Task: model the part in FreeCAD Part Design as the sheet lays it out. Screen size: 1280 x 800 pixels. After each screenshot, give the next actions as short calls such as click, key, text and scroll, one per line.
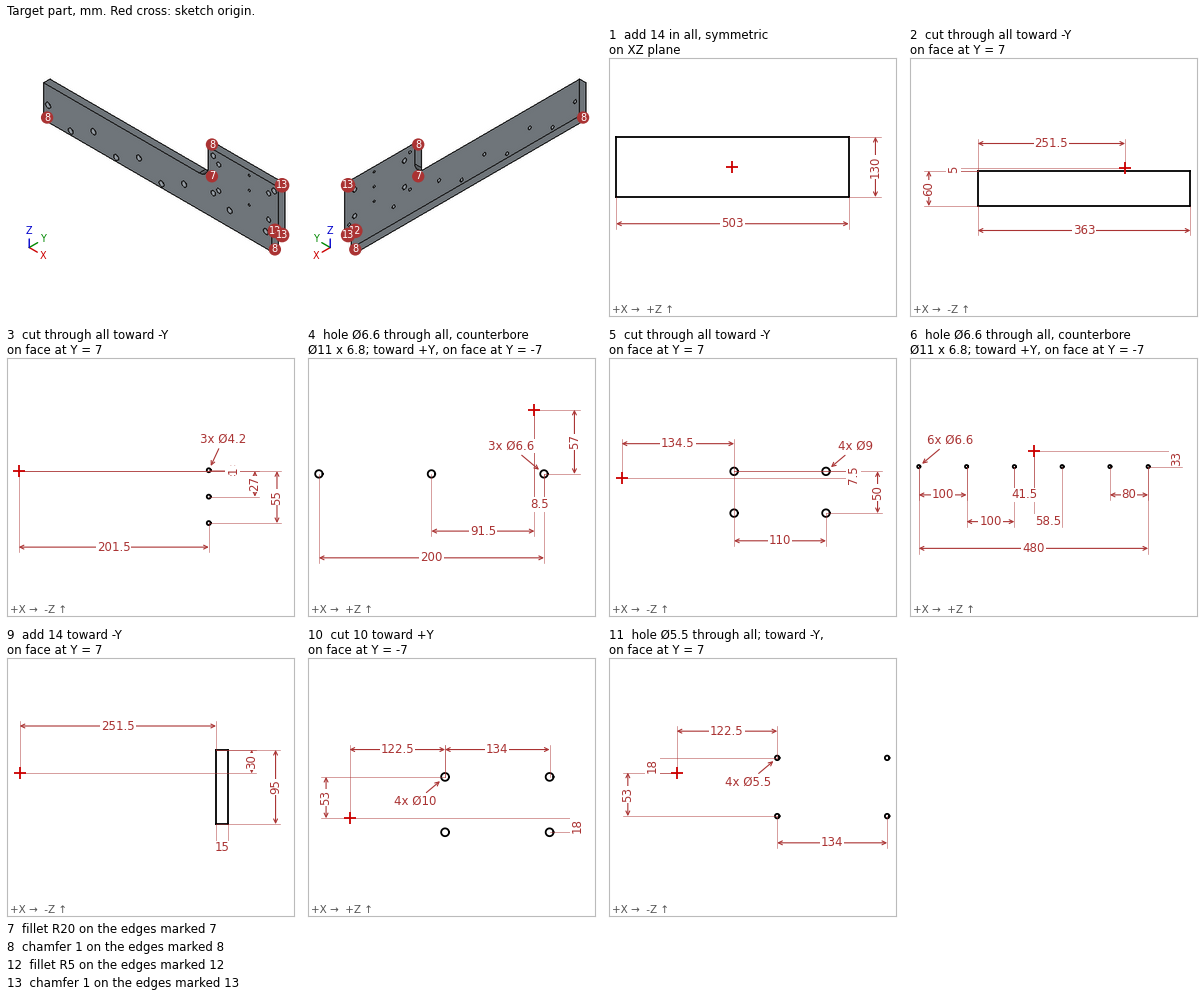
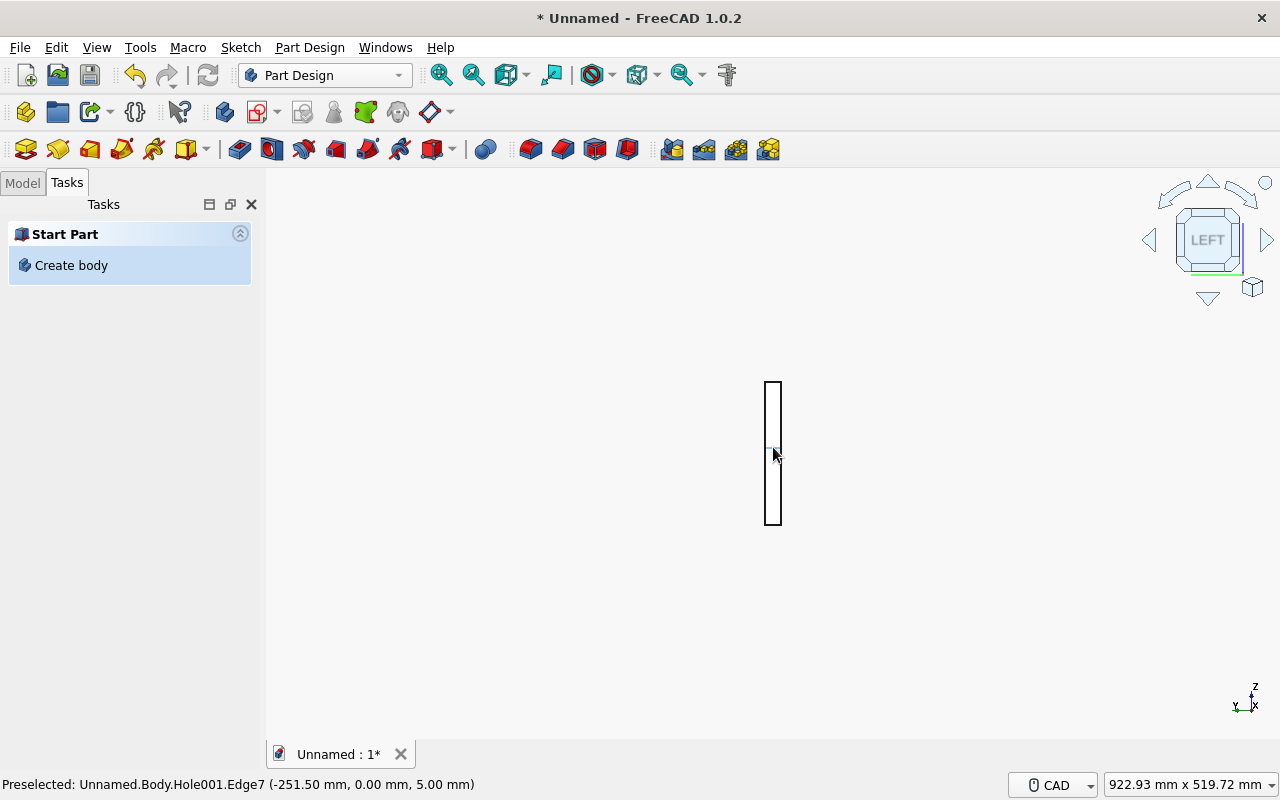
key(v)
key(3)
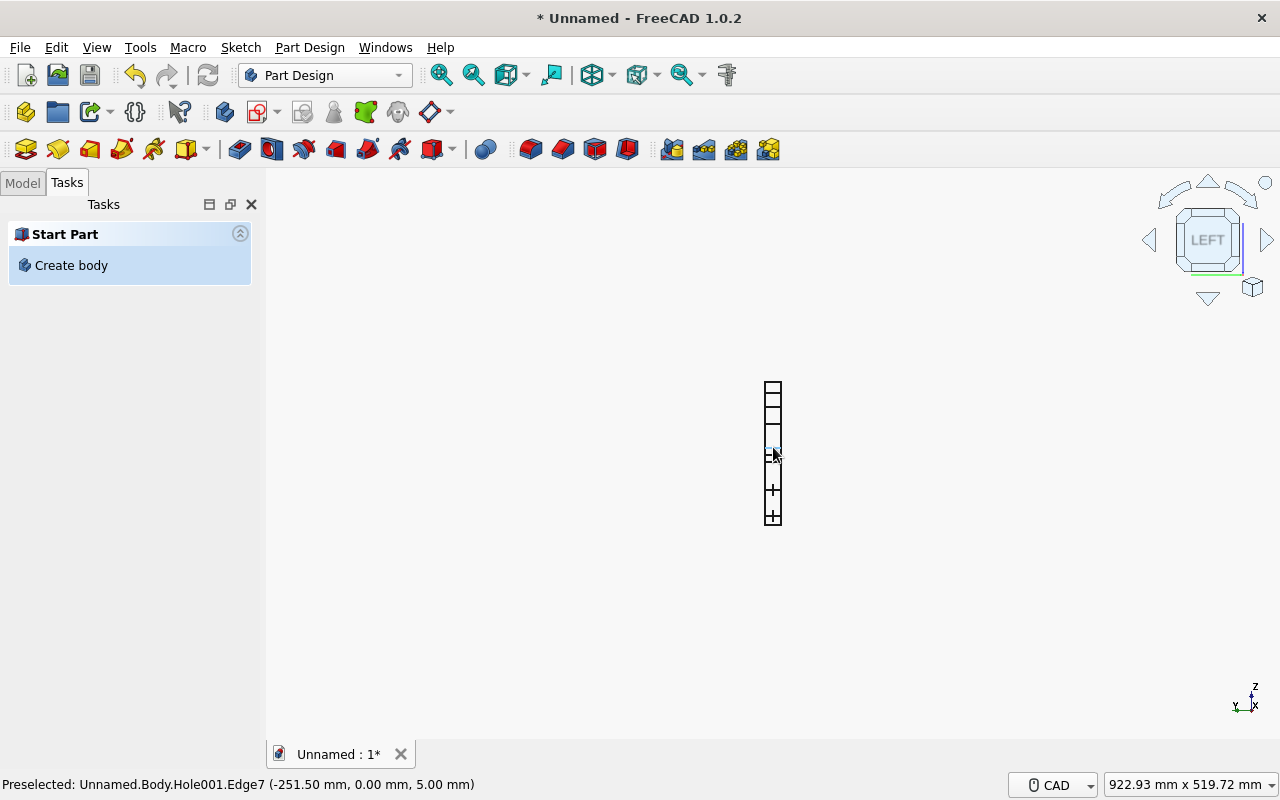
key(0)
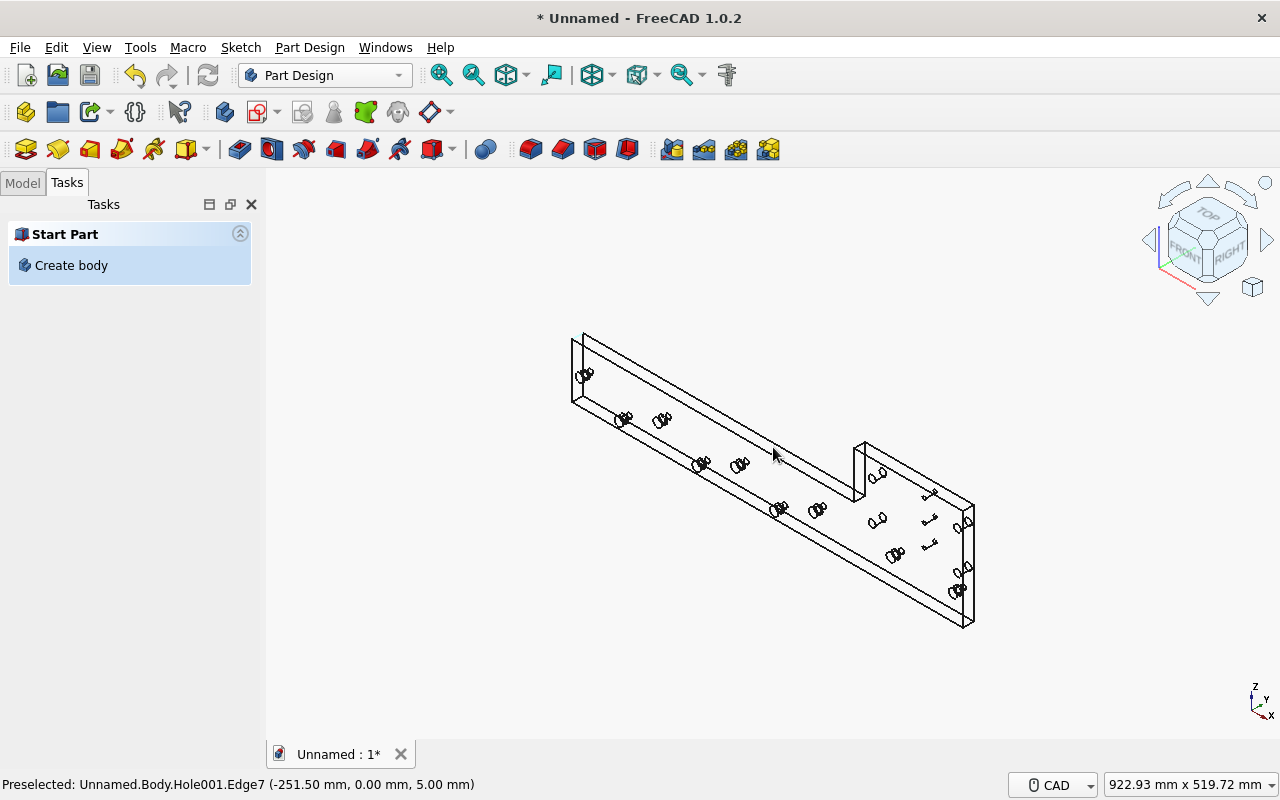
click(861, 497)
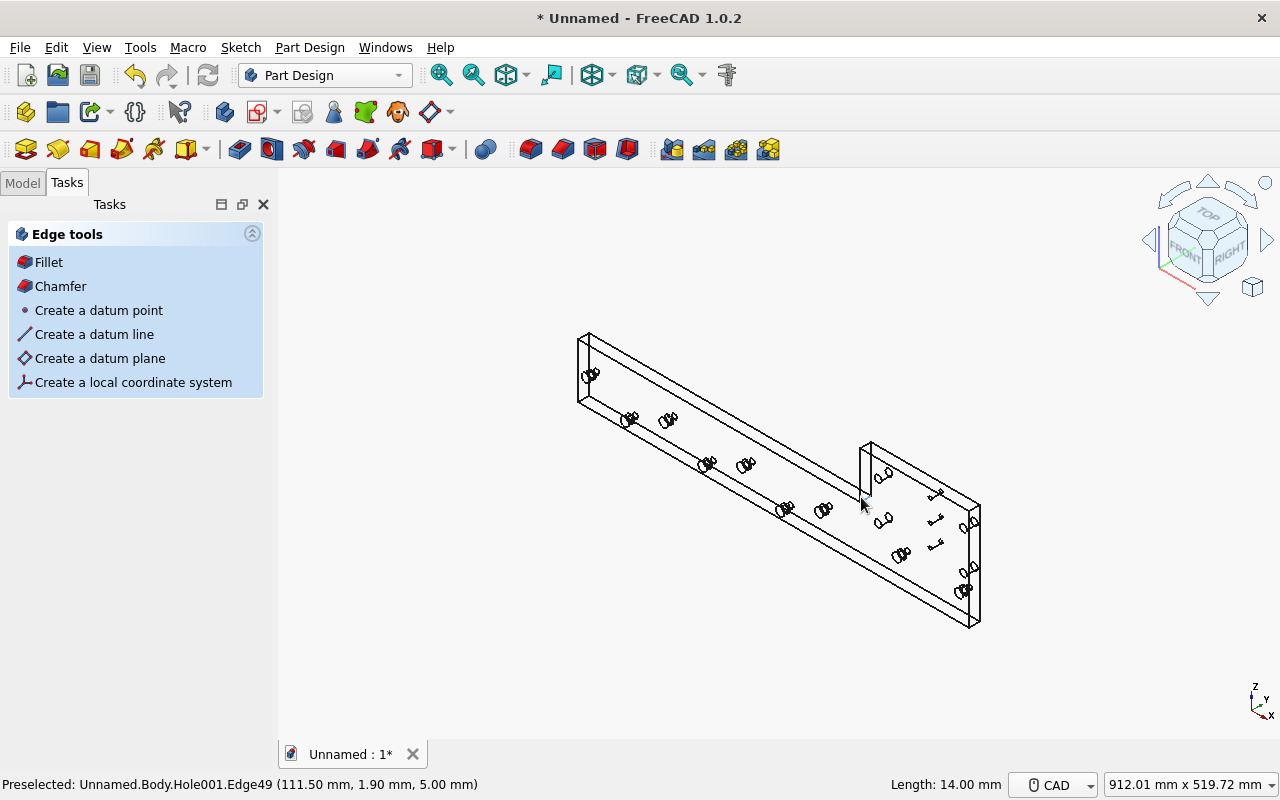
key(v)
key(1)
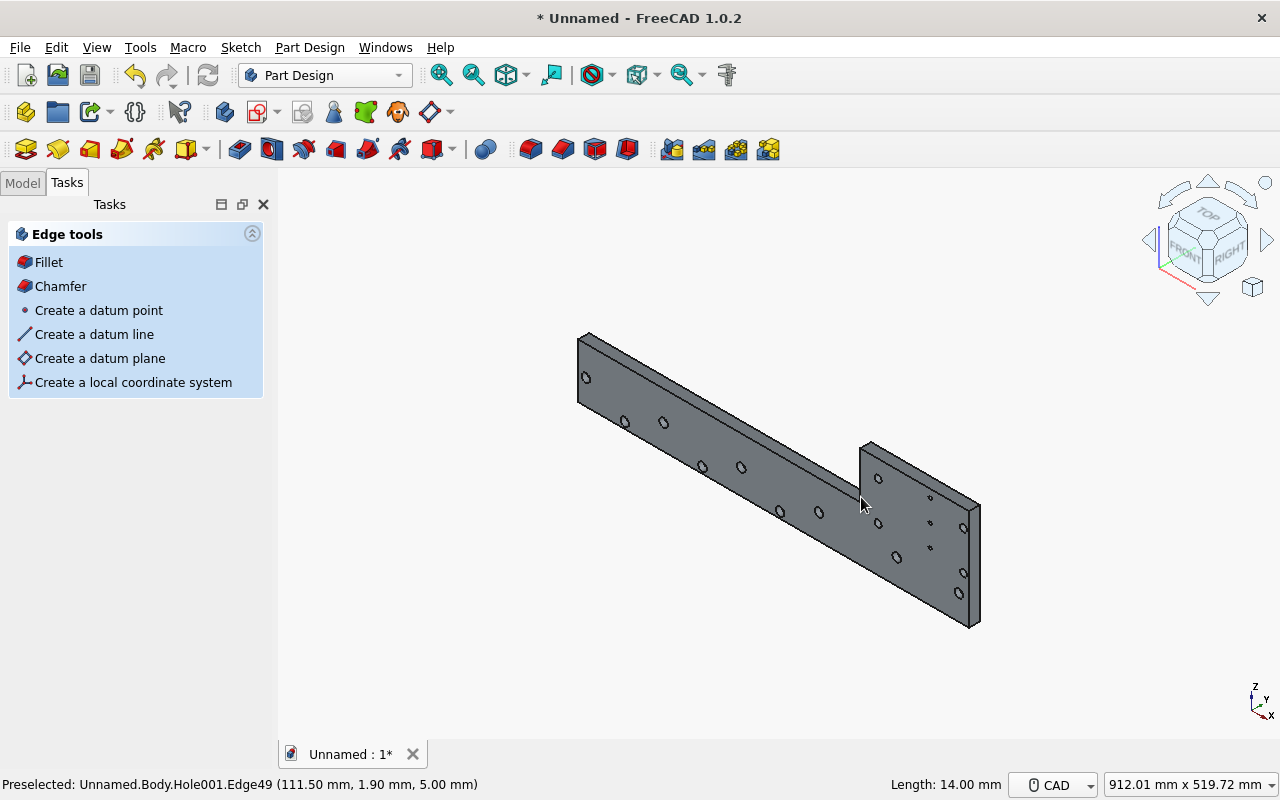
click(532, 150)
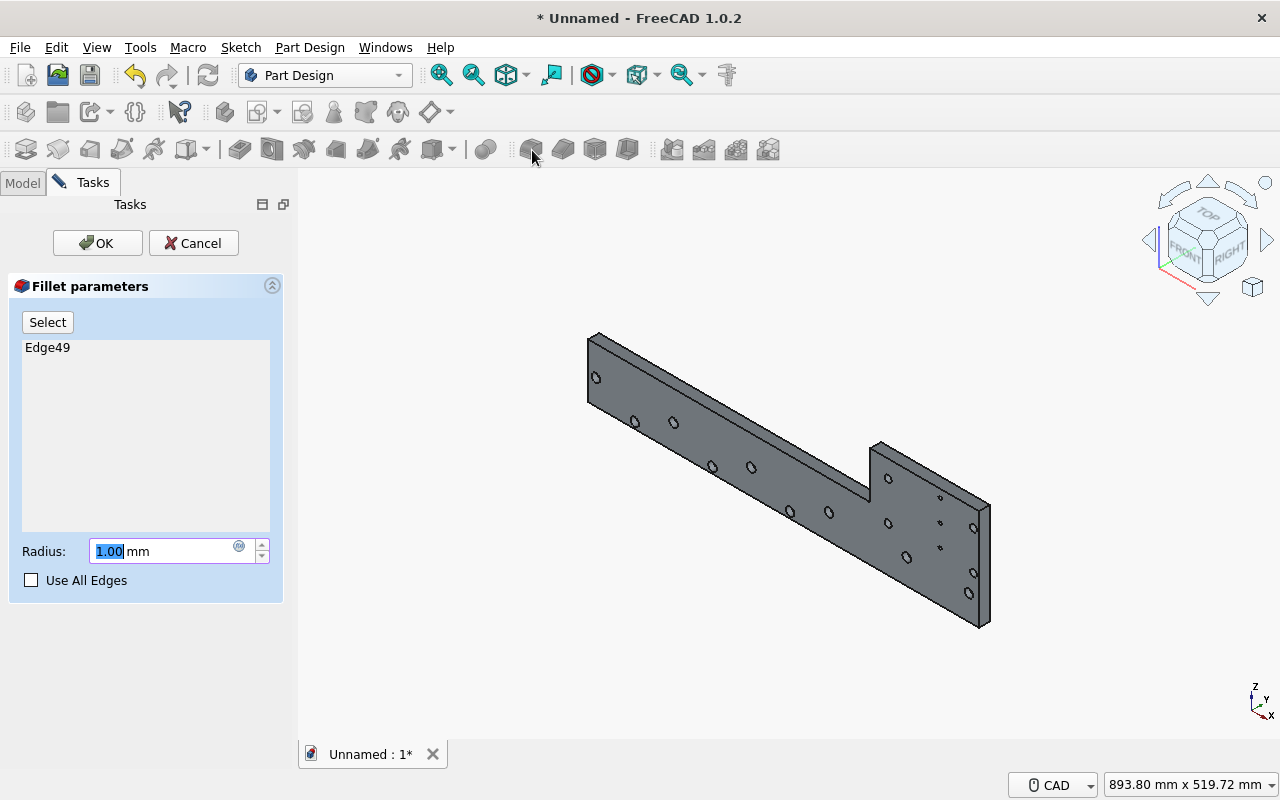
text(20)
key(Tab)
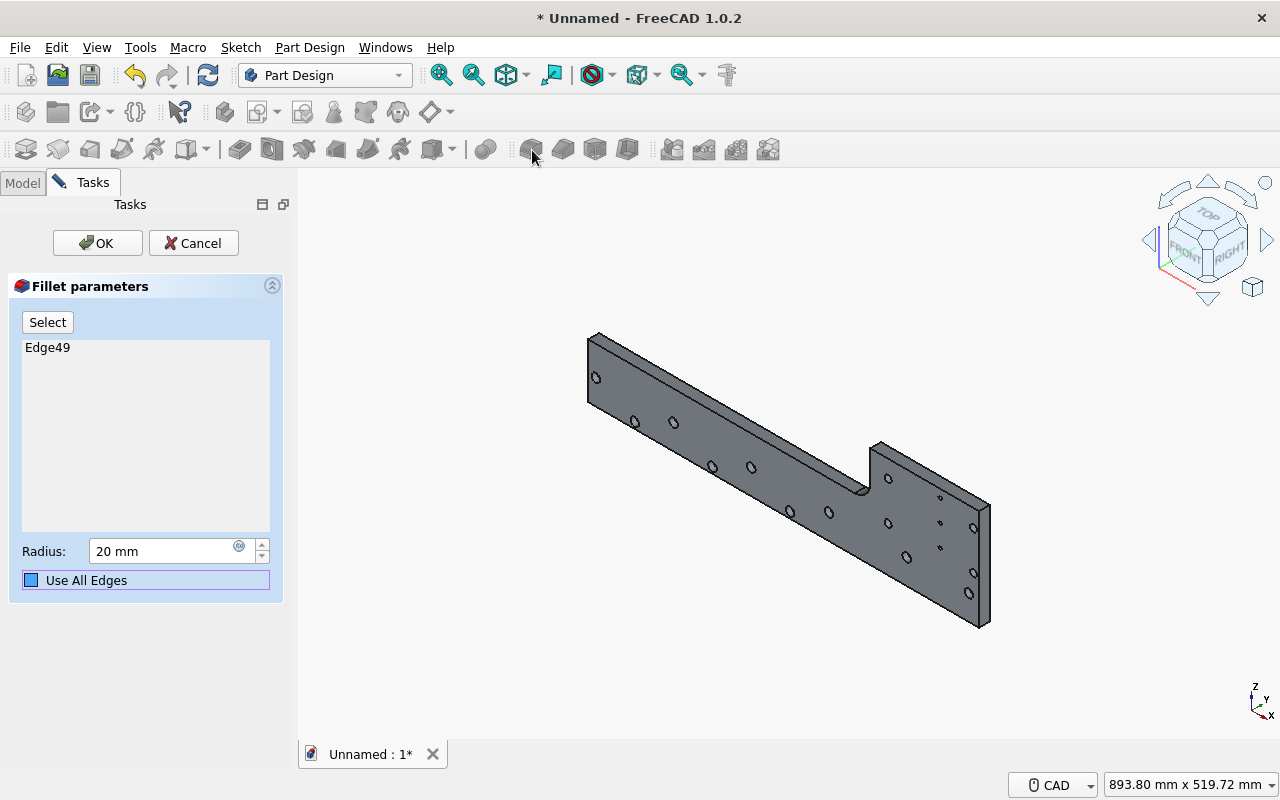
click(98, 243)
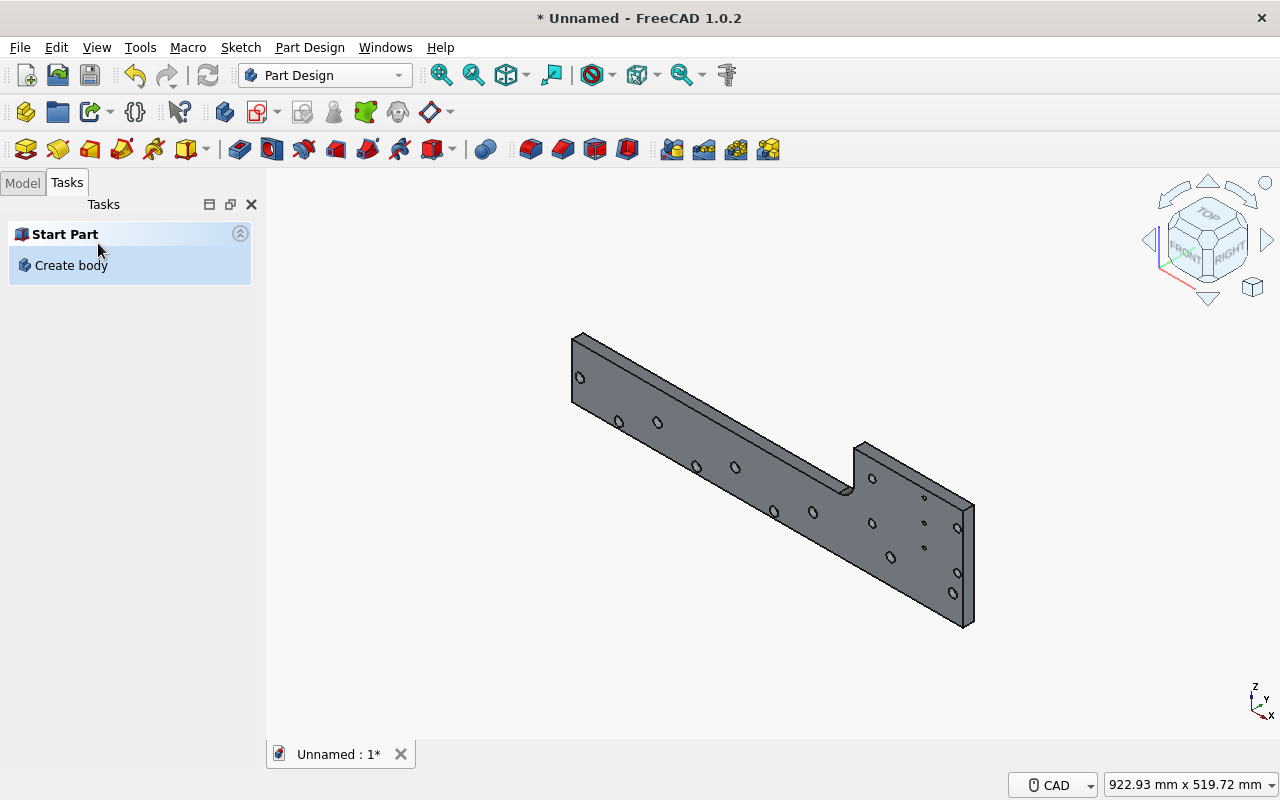
scroll(860, 444, up, 5)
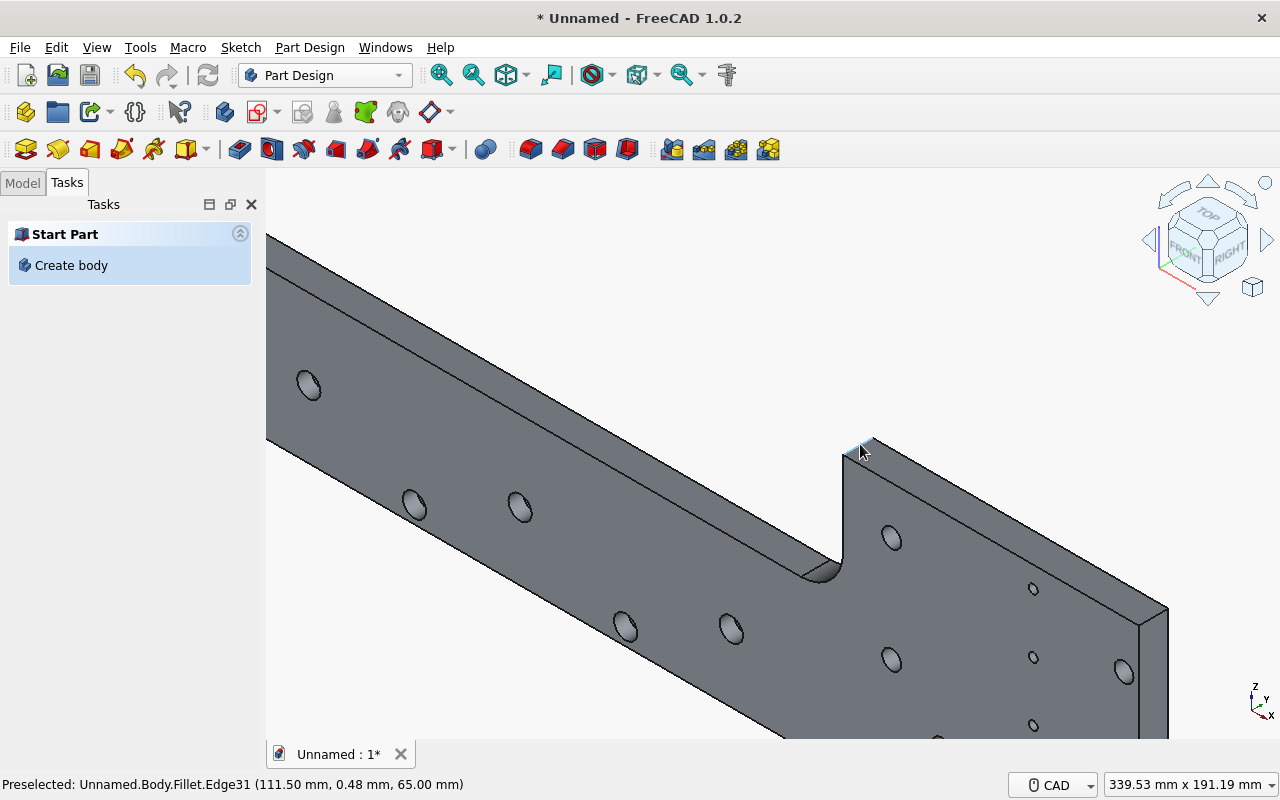
click(442, 76)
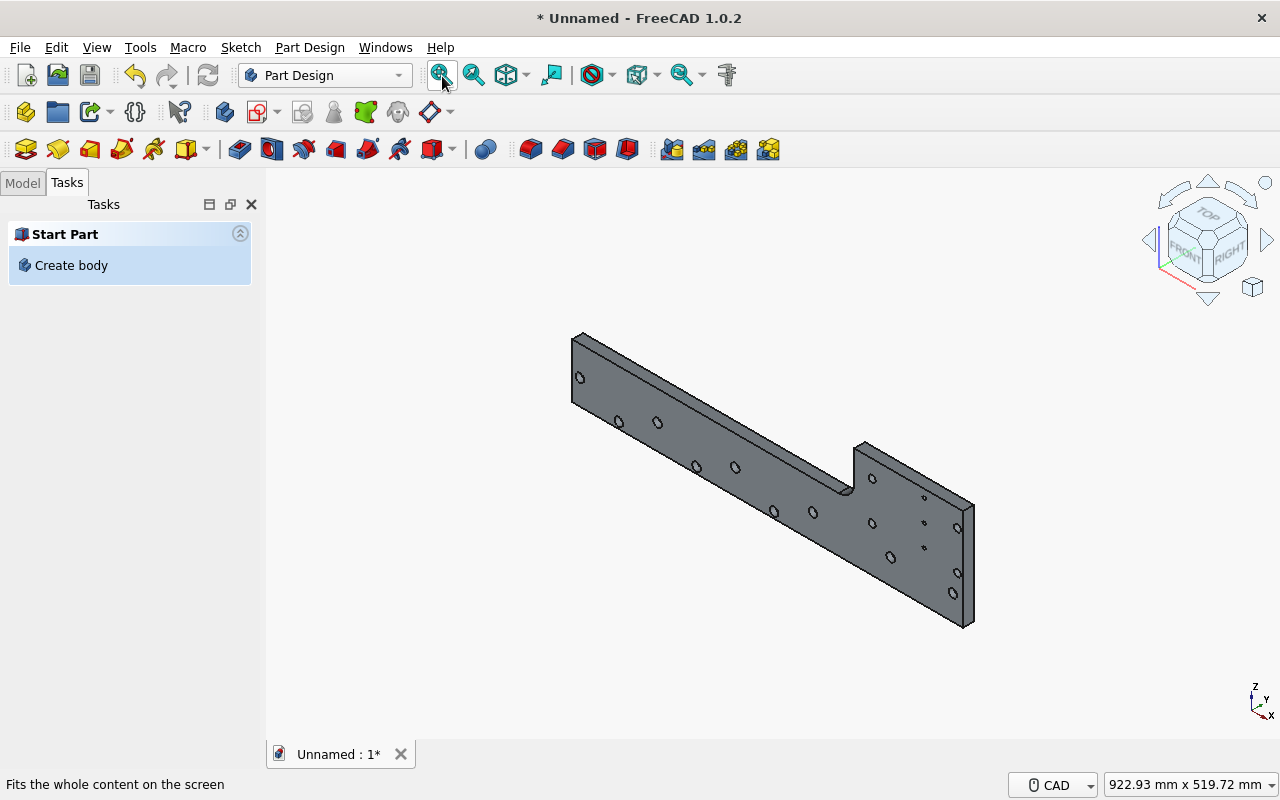
key(2)